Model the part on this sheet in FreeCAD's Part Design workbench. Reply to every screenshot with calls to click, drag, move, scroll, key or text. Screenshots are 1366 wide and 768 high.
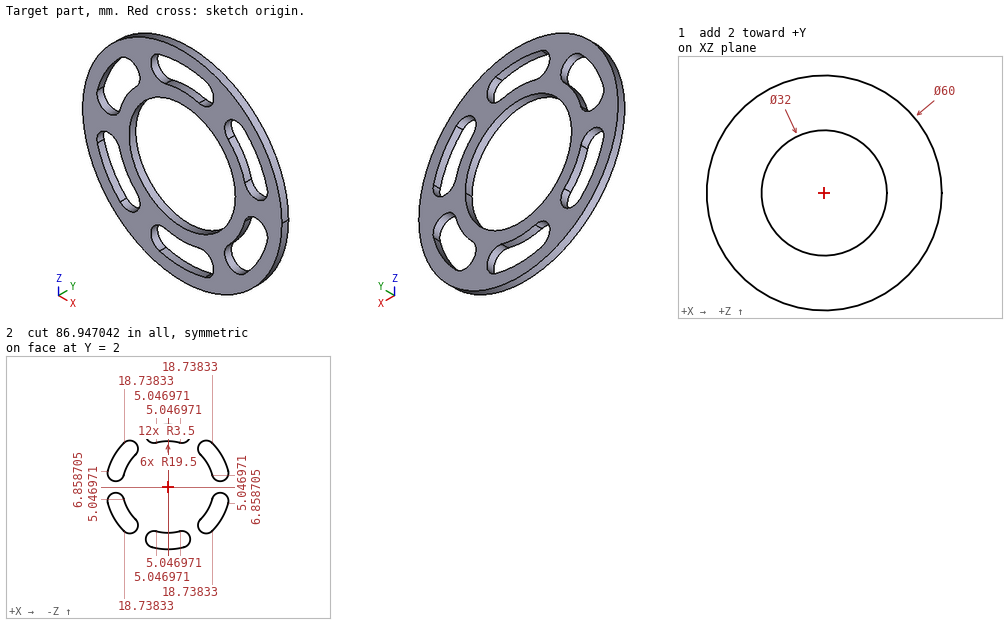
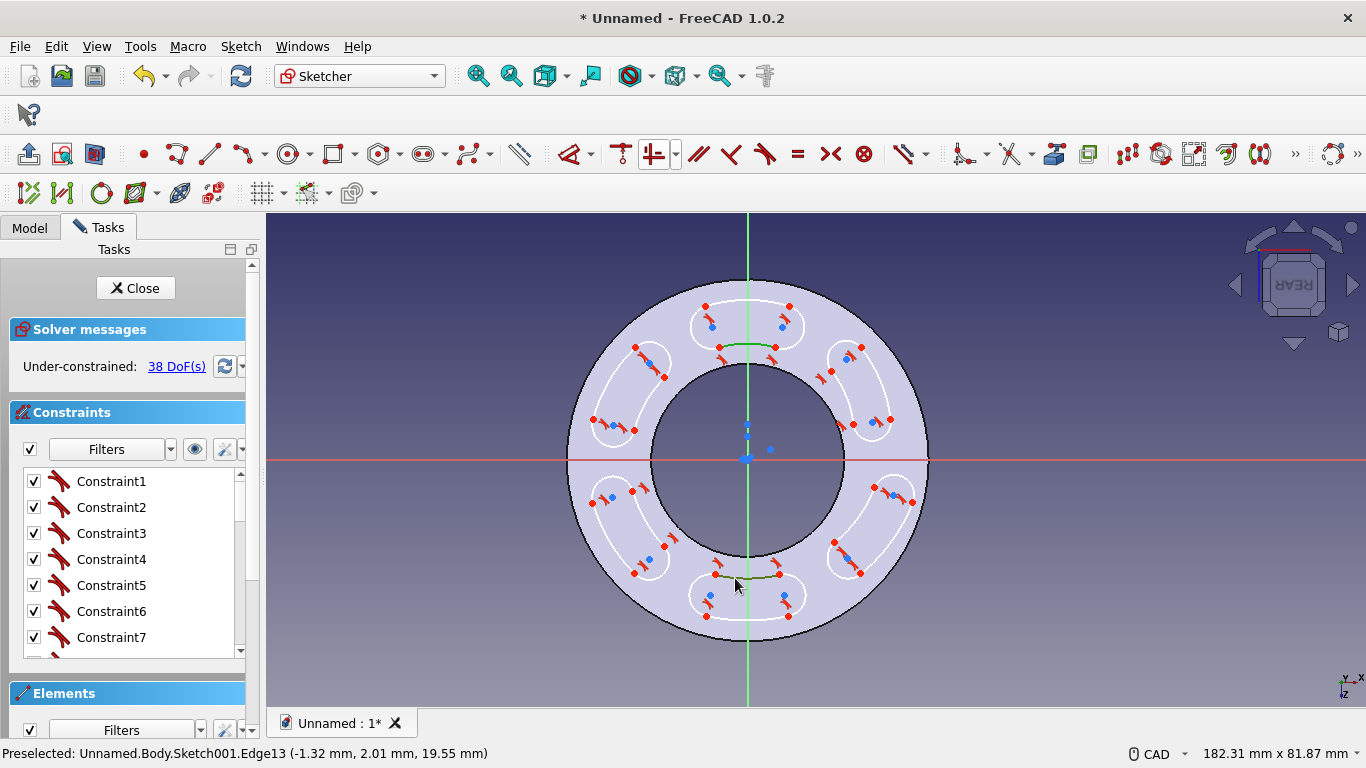
click(621, 154)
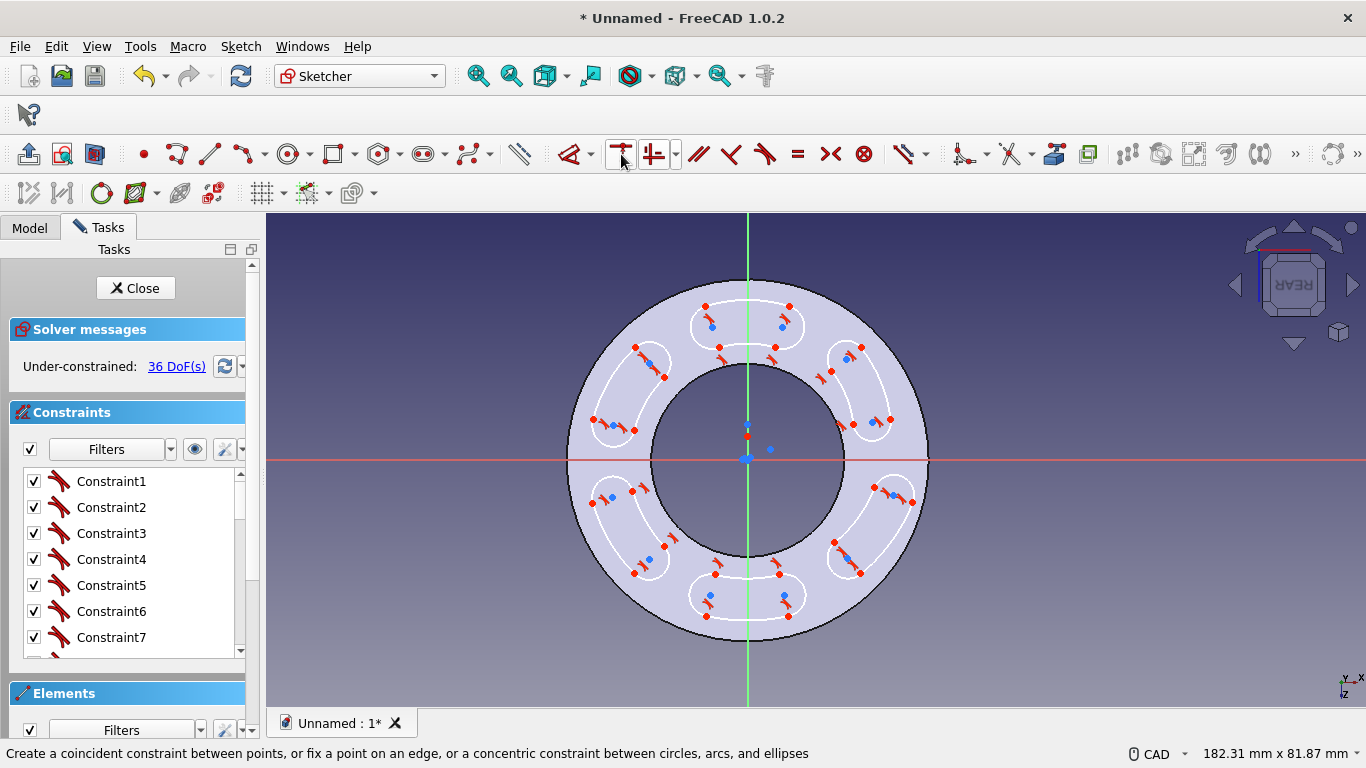
click(759, 344)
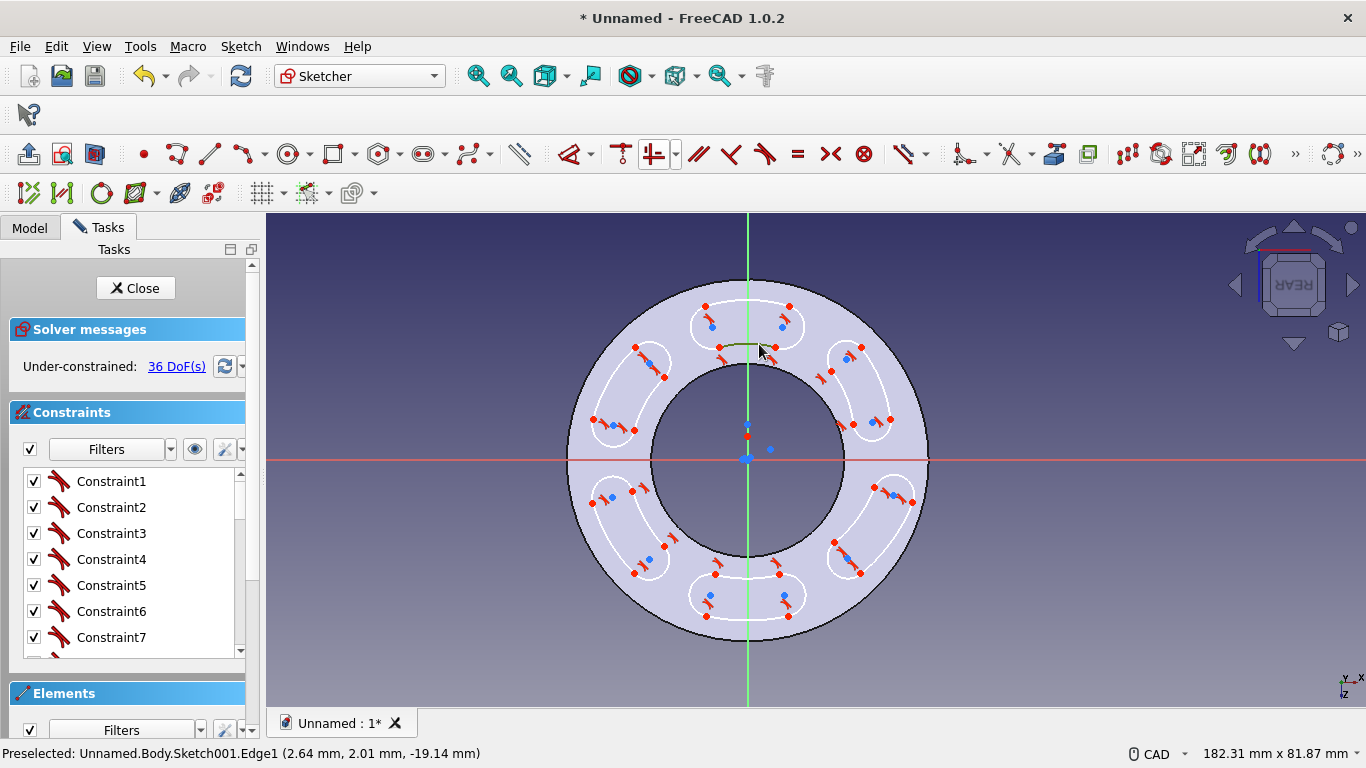
click(731, 620)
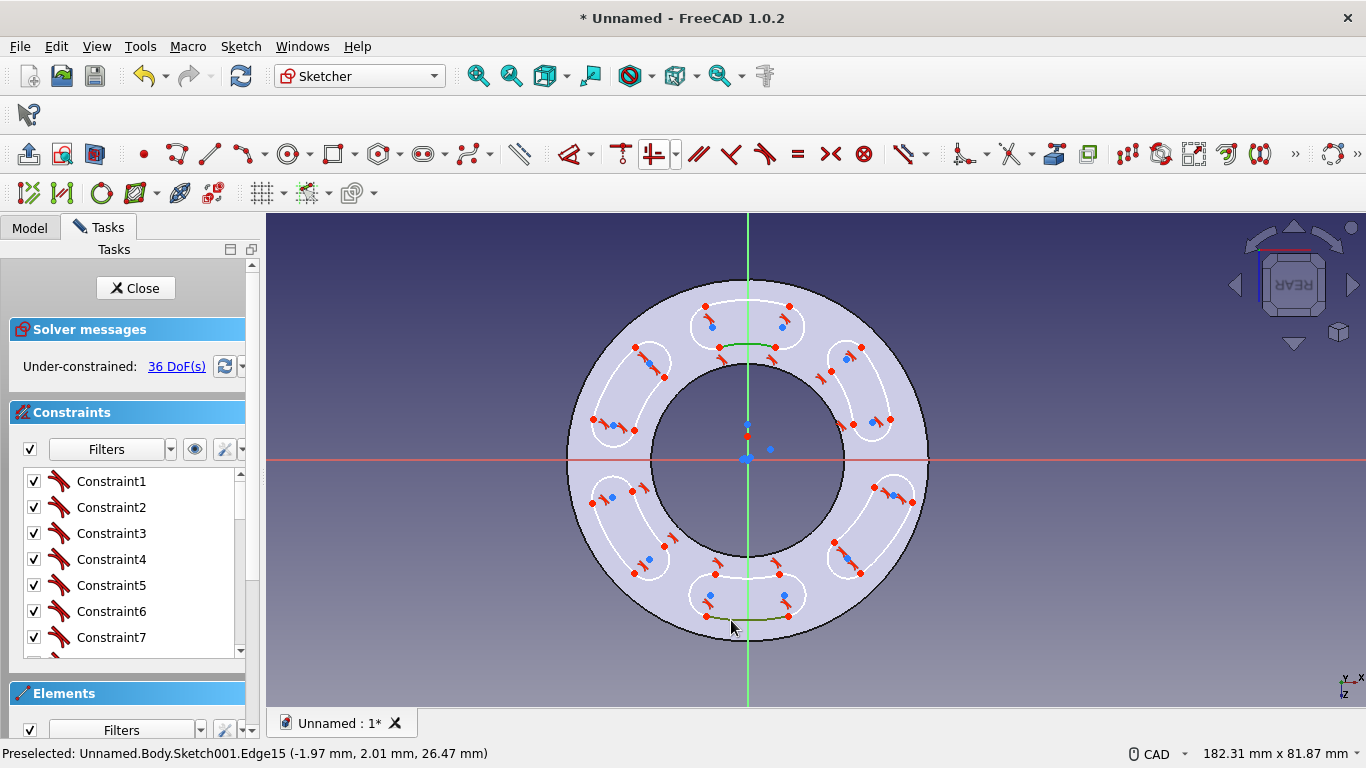
click(621, 154)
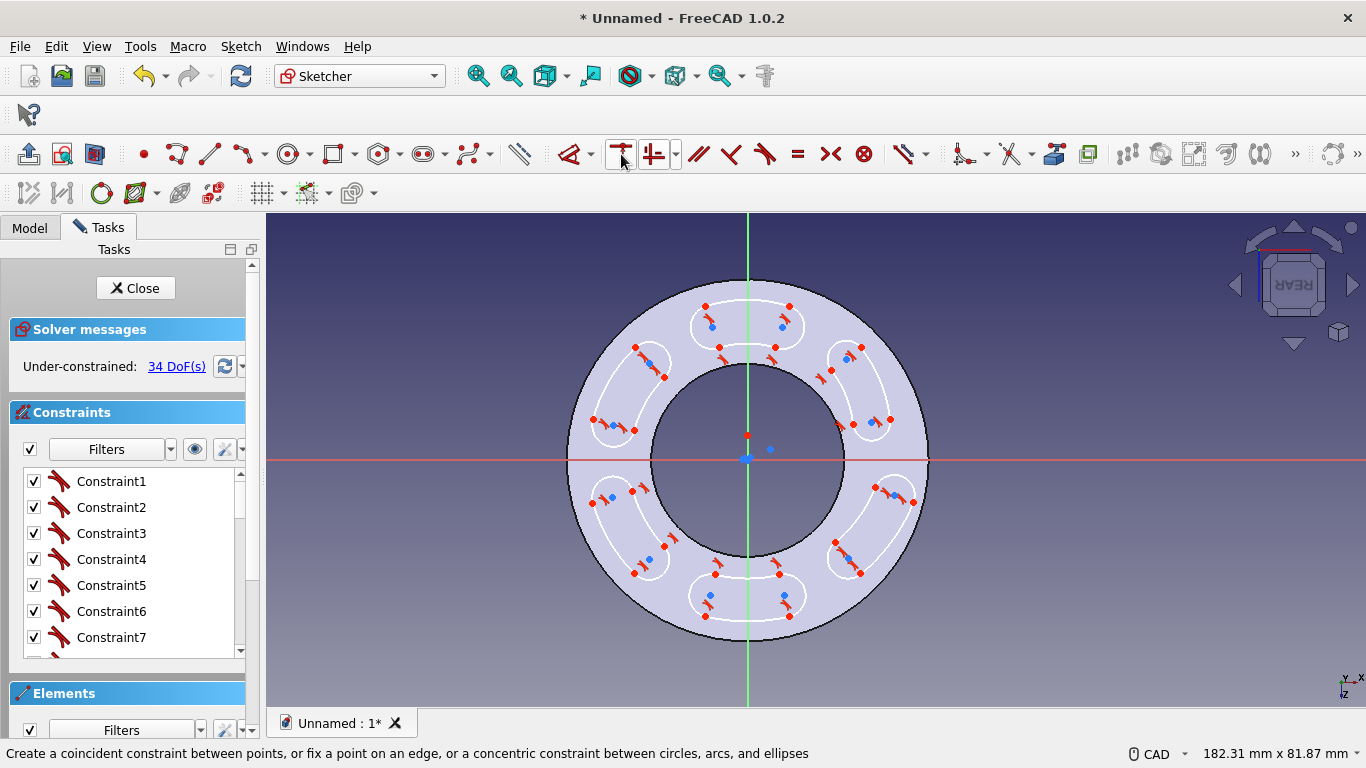
click(759, 344)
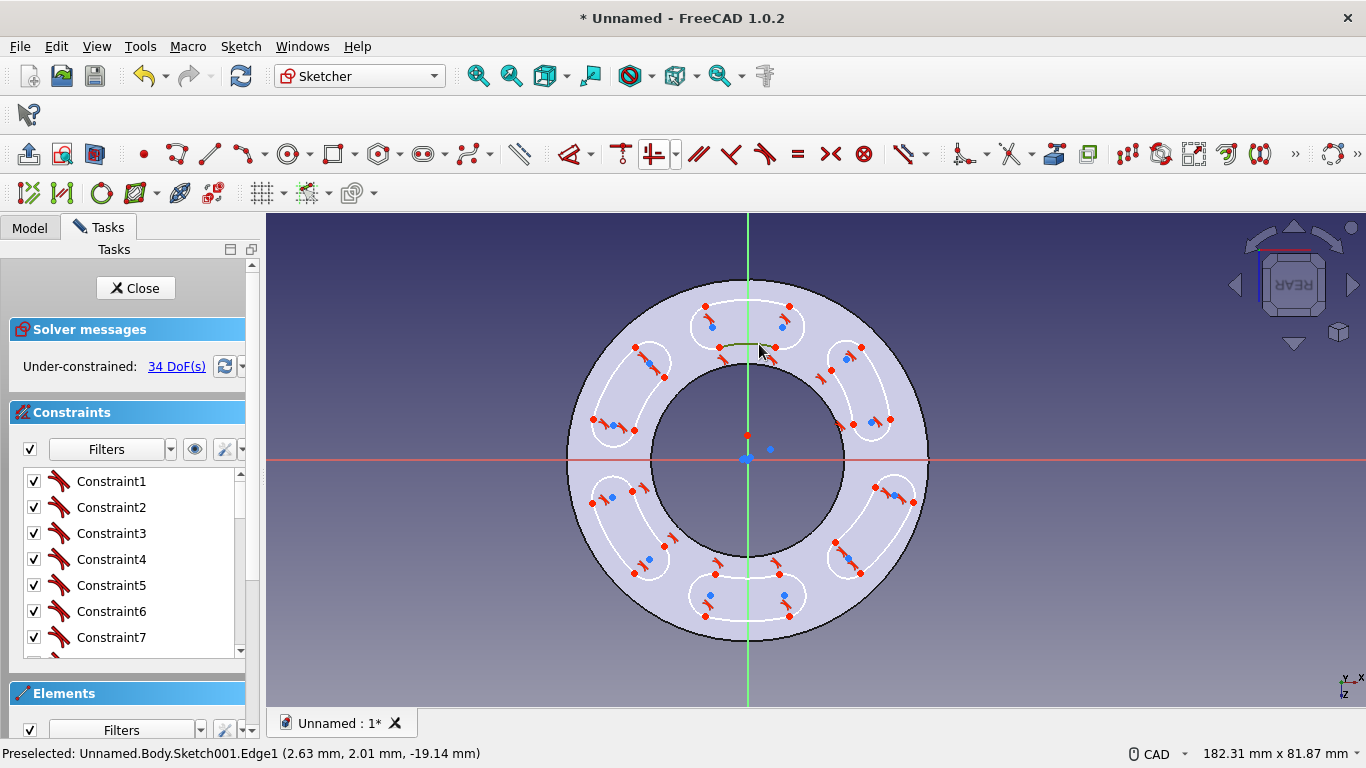
click(640, 509)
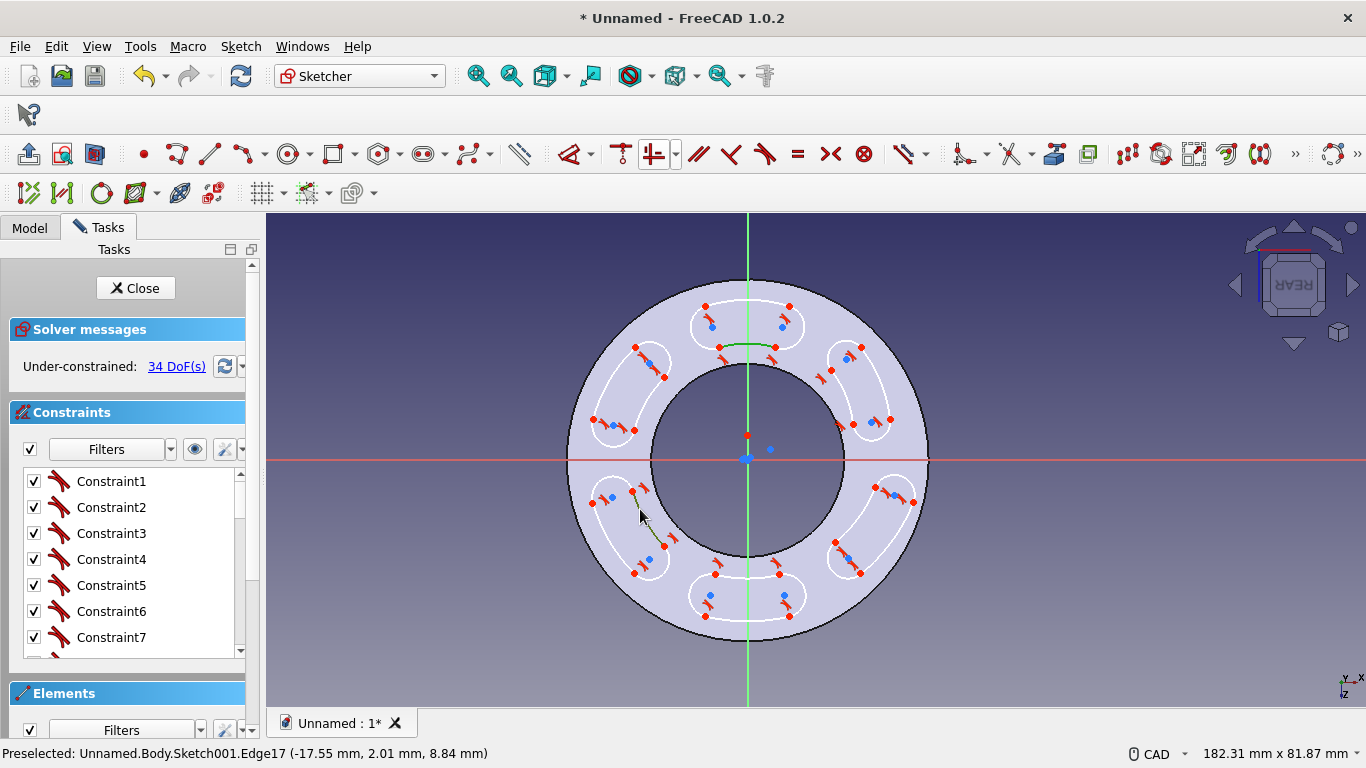
click(621, 154)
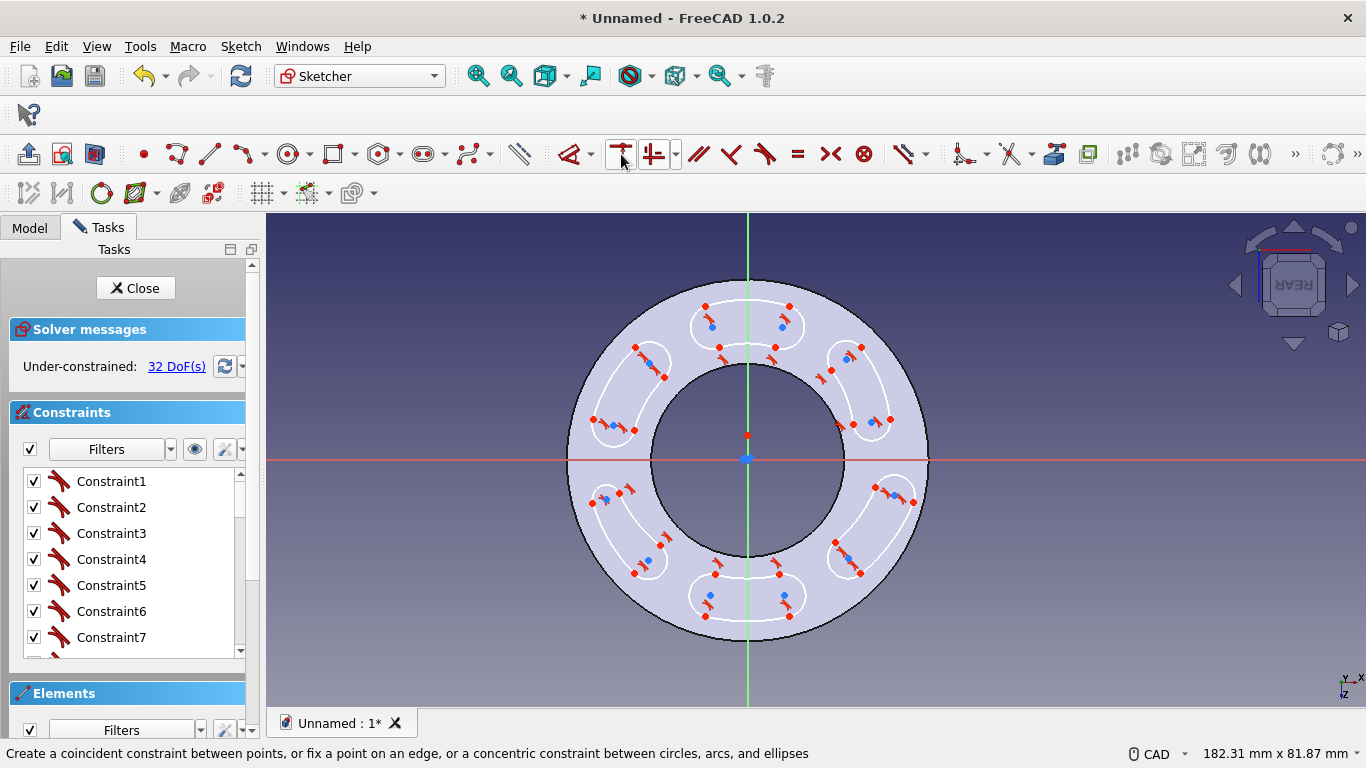
click(759, 344)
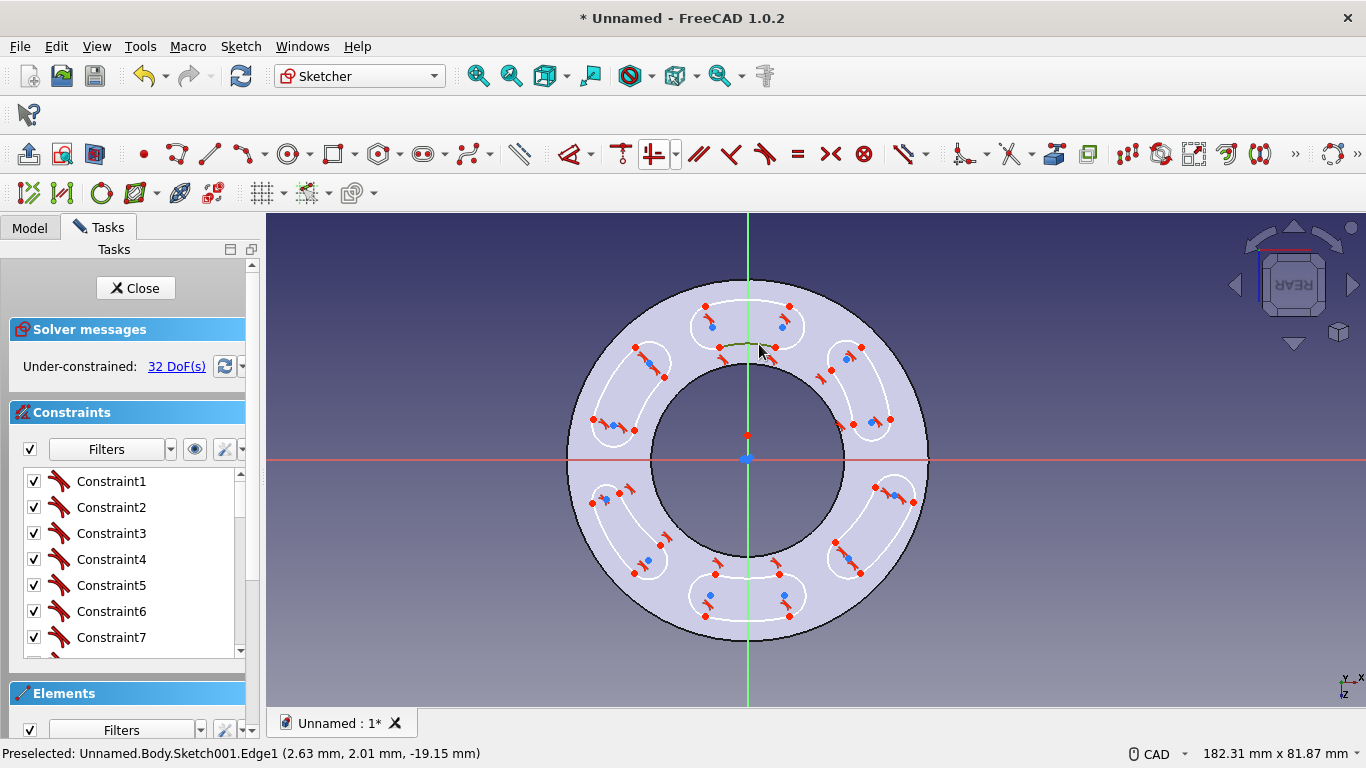
click(602, 526)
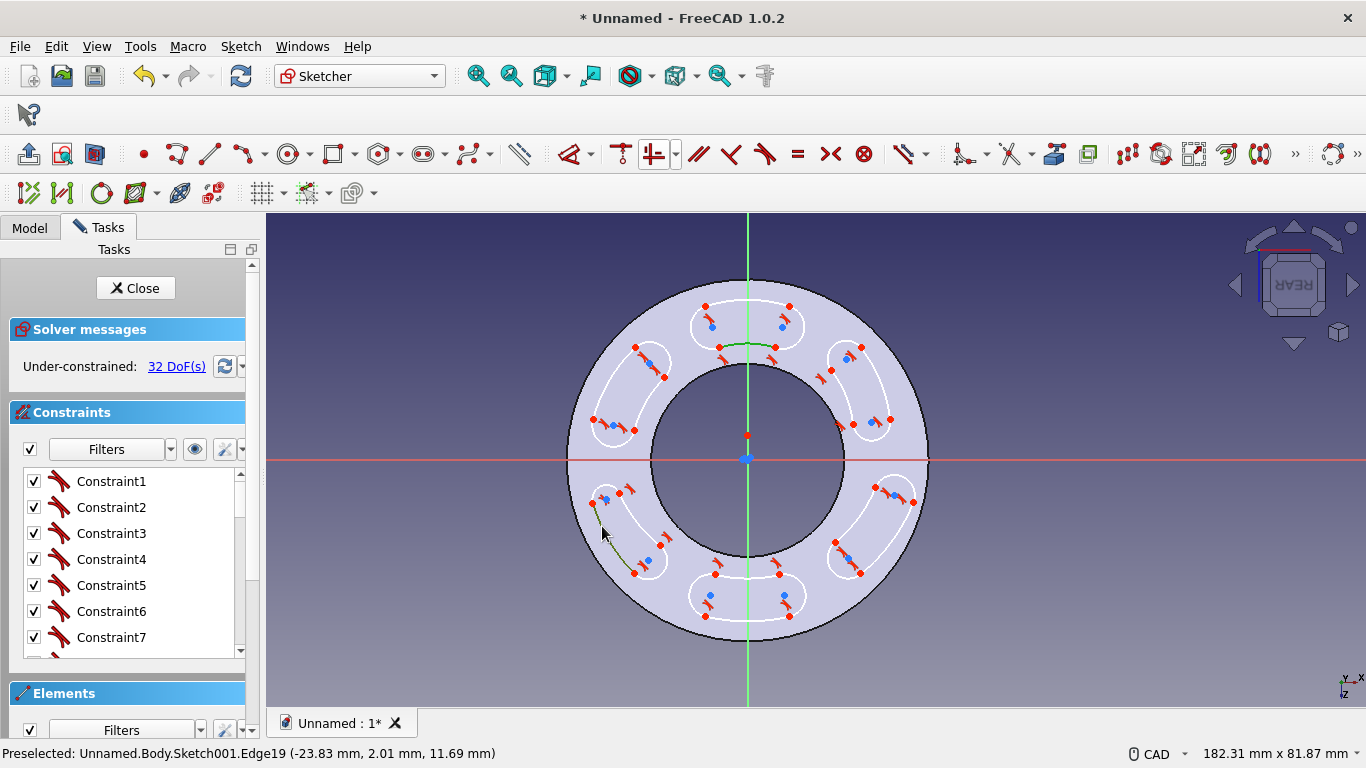
click(621, 154)